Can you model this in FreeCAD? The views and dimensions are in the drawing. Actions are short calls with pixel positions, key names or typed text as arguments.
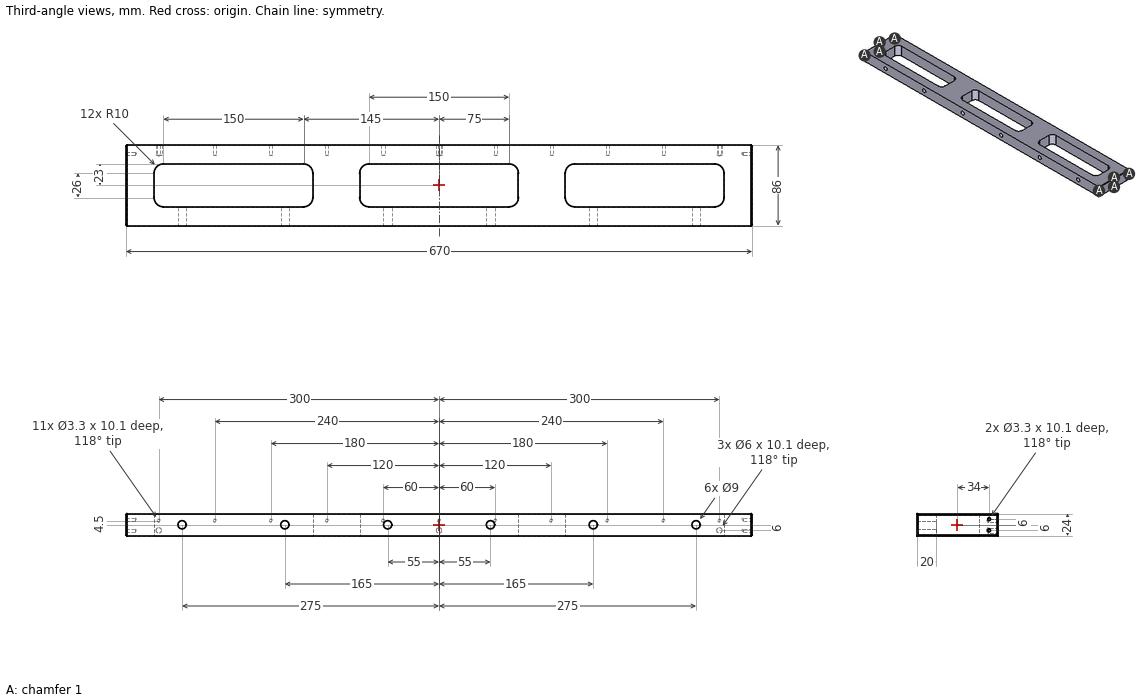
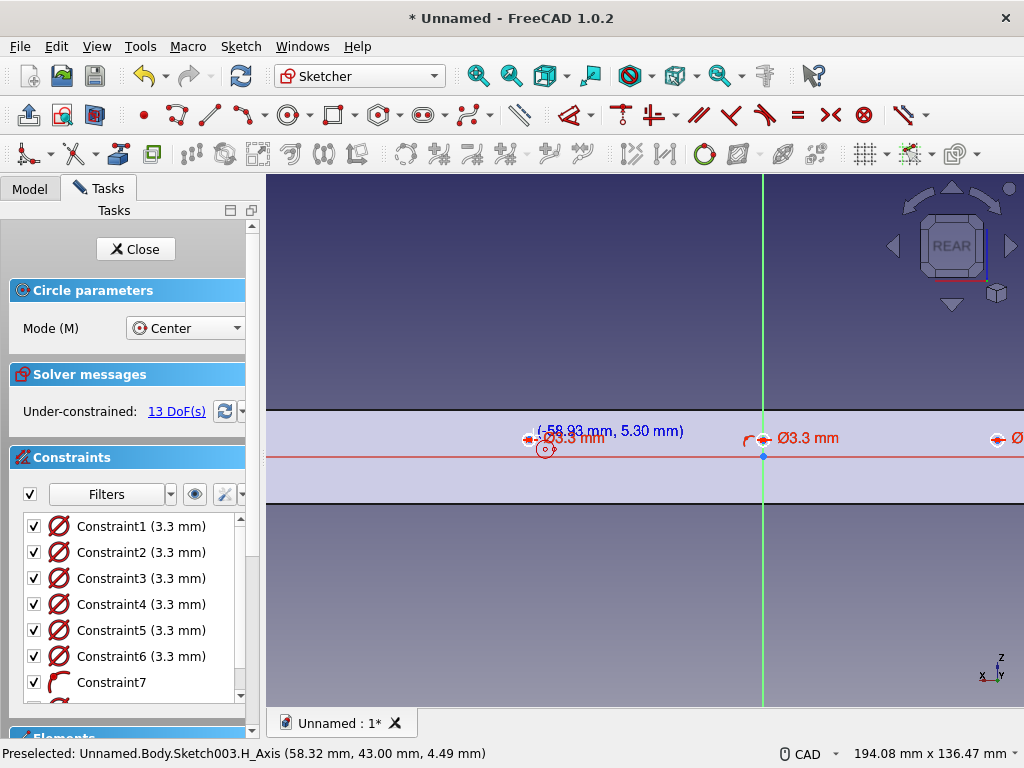
scroll(294, 439, up, 7)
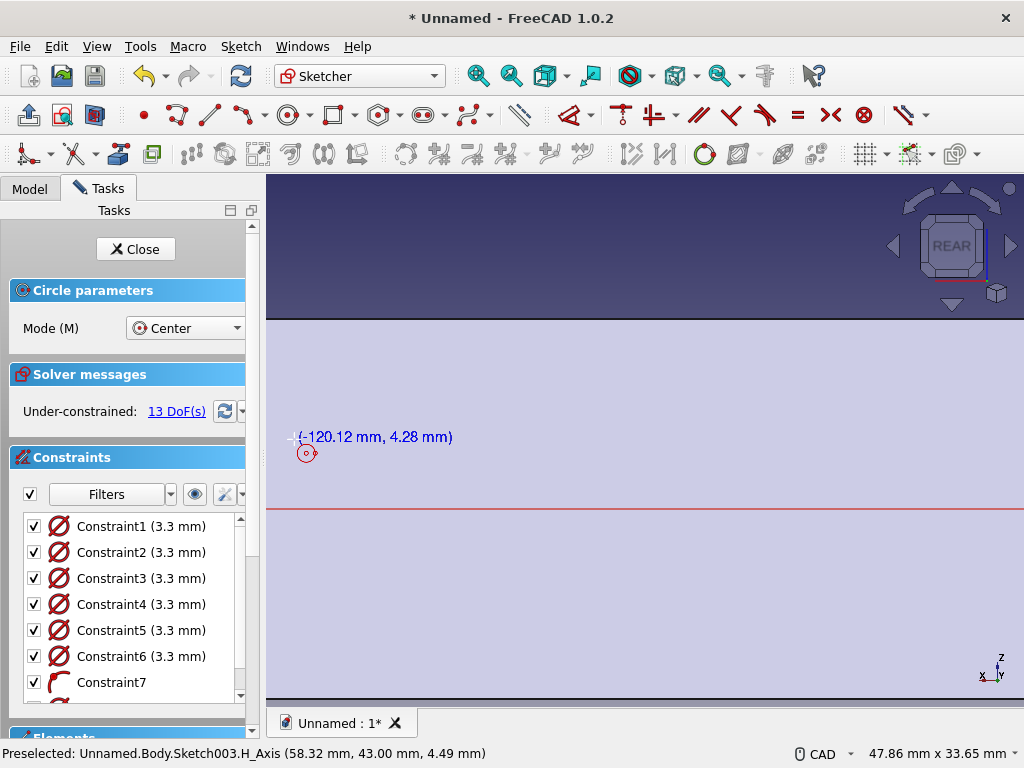
scroll(492, 439, down, 15)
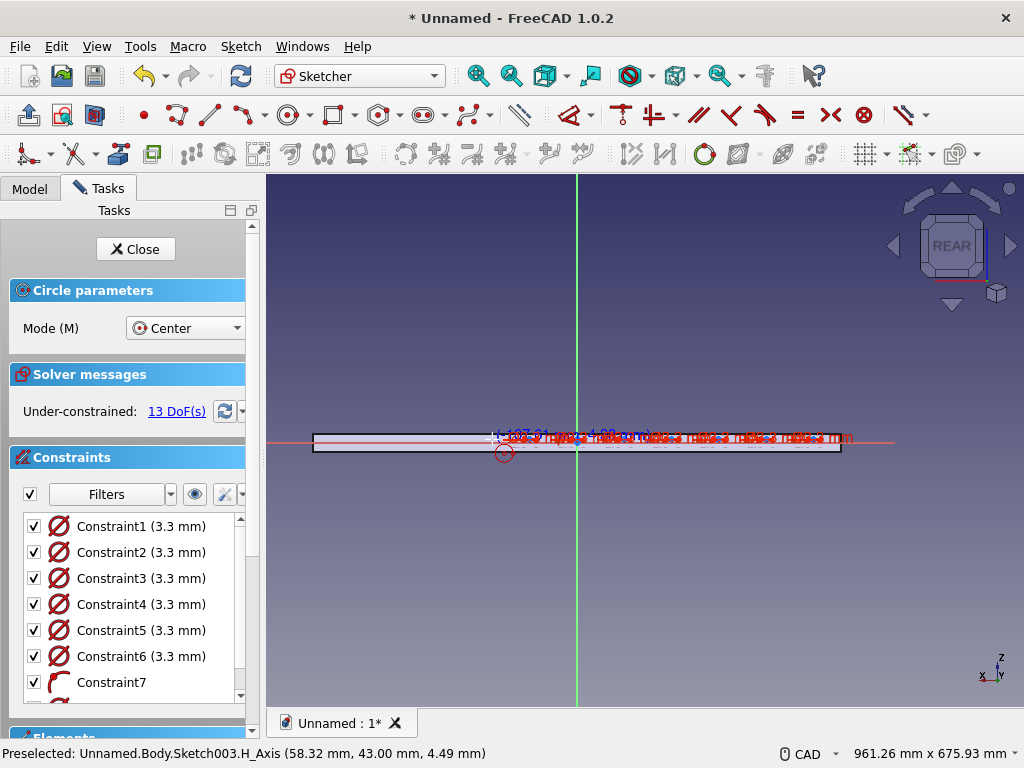
scroll(483, 439, up, 8)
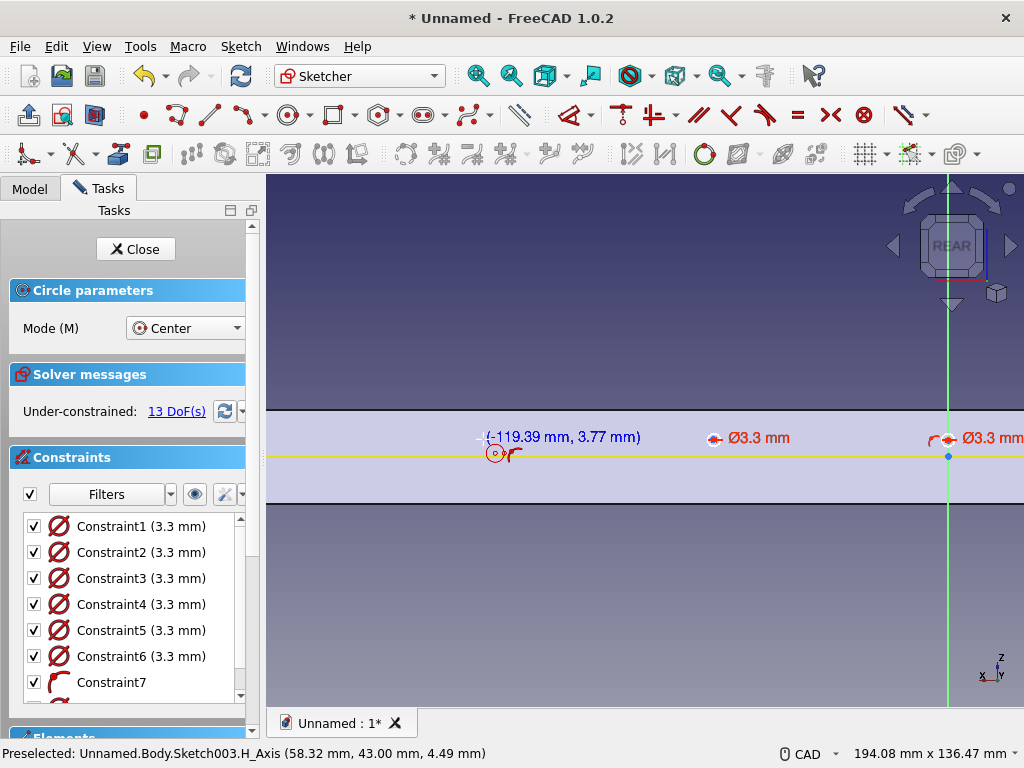
click(479, 439)
move(484, 435)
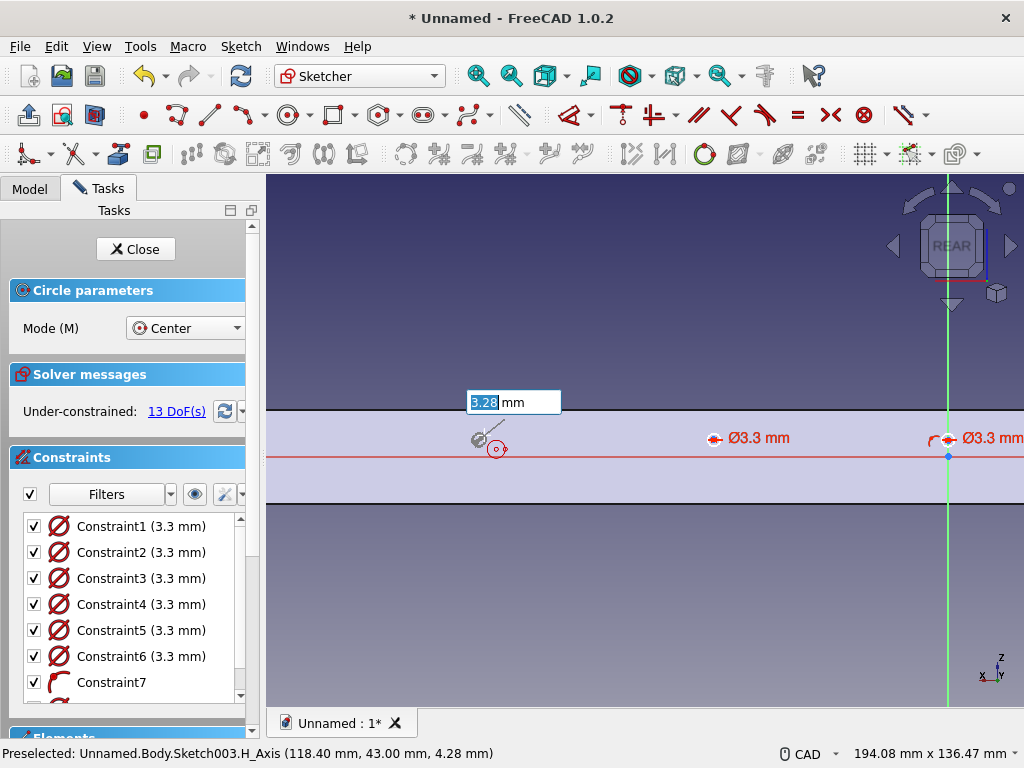
text(3.3)
key(Return)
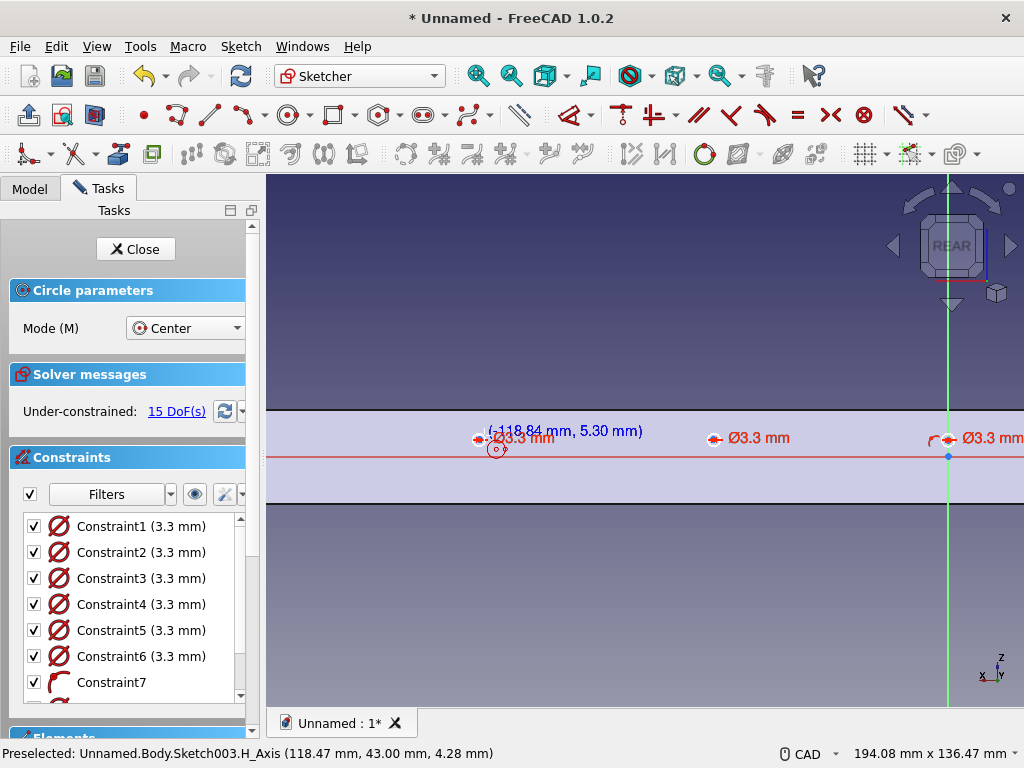
scroll(503, 440, down, 9)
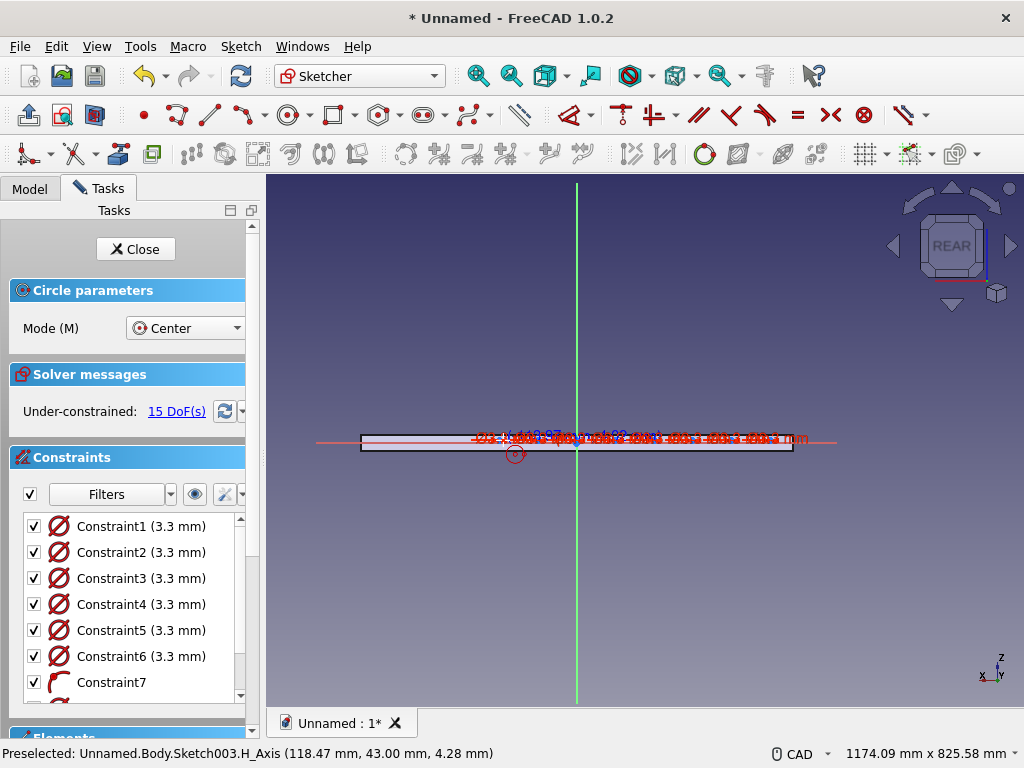
scroll(461, 440, up, 16)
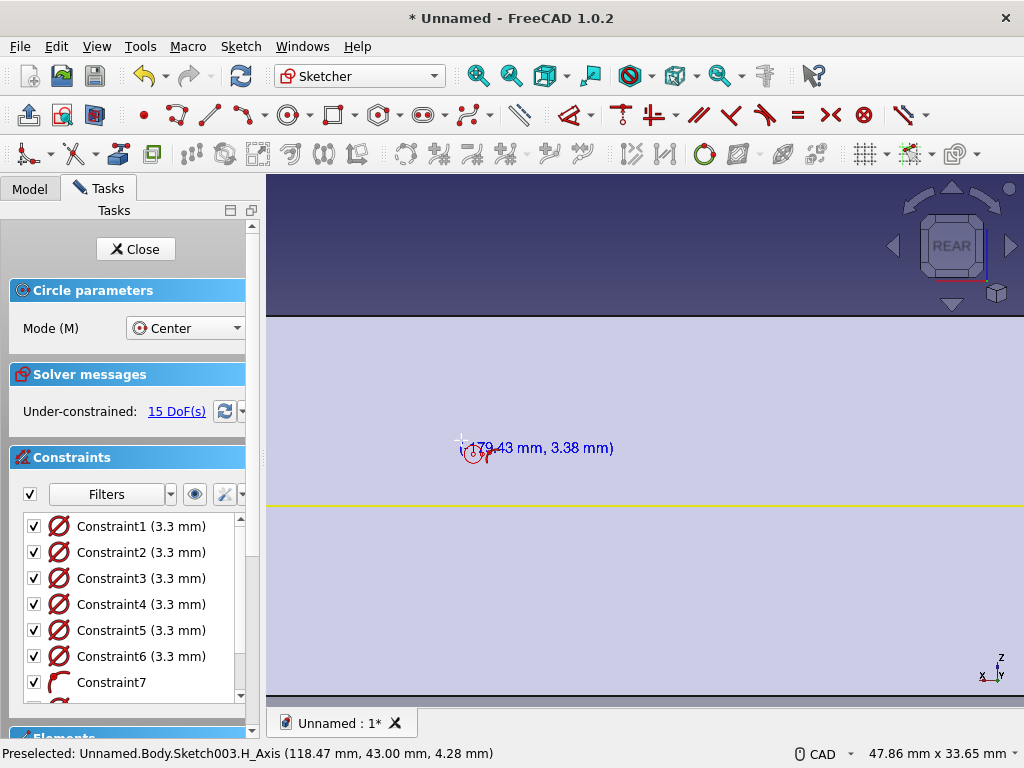
scroll(434, 440, down, 15)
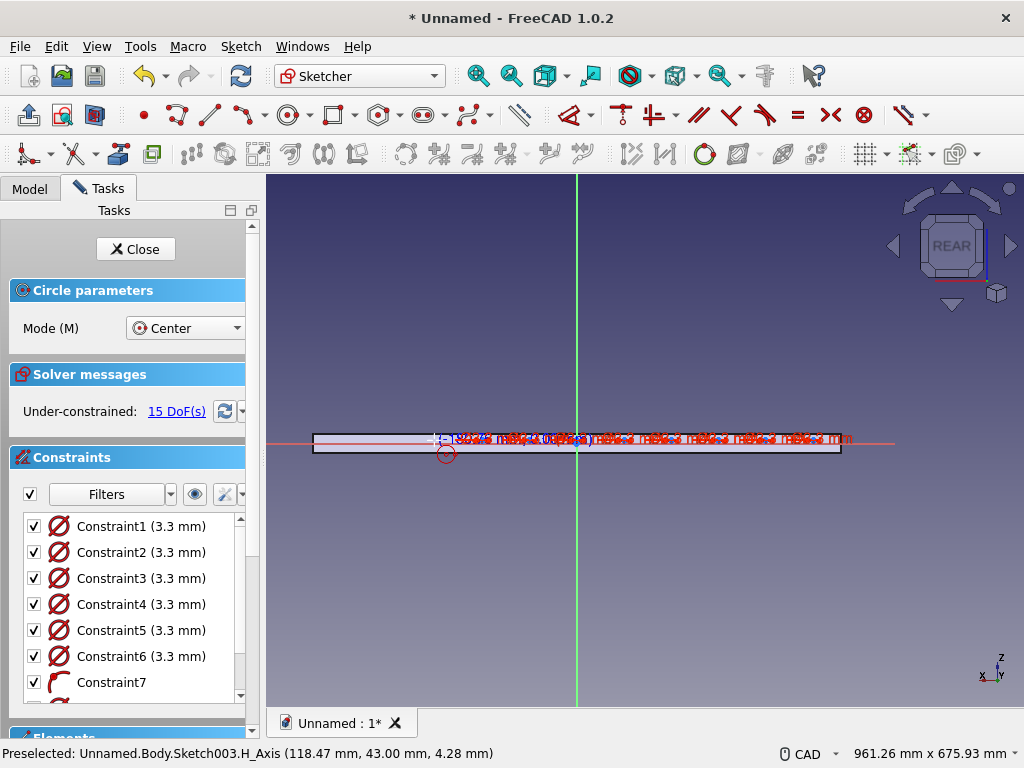
scroll(435, 440, up, 8)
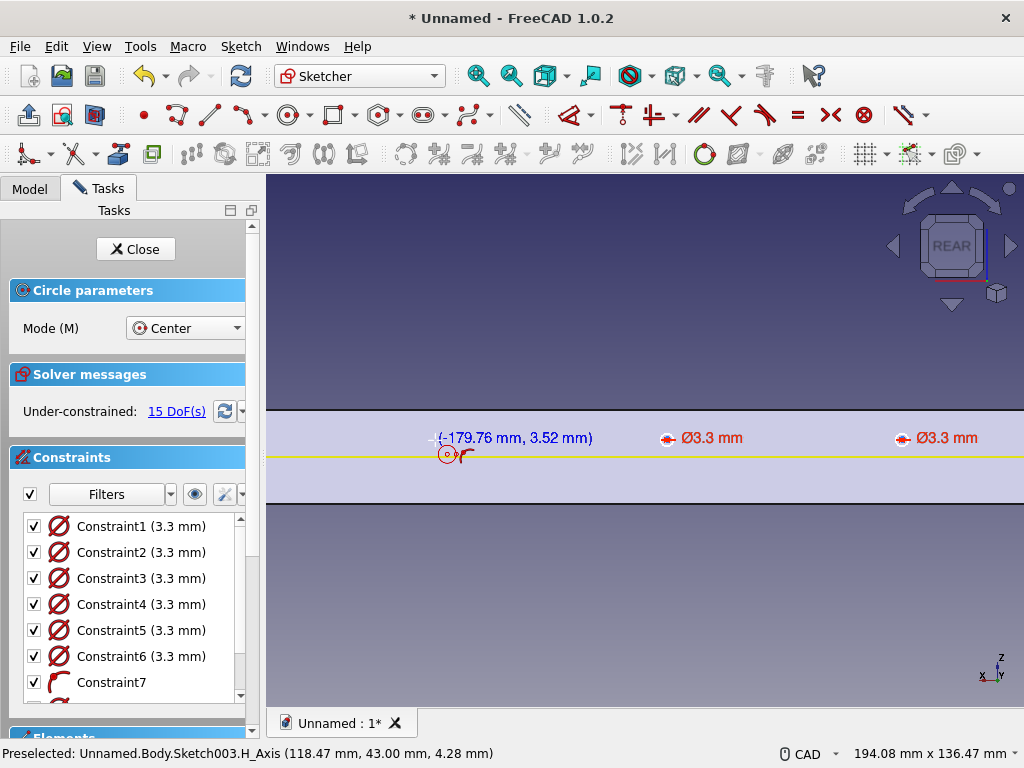
click(433, 439)
move(438, 435)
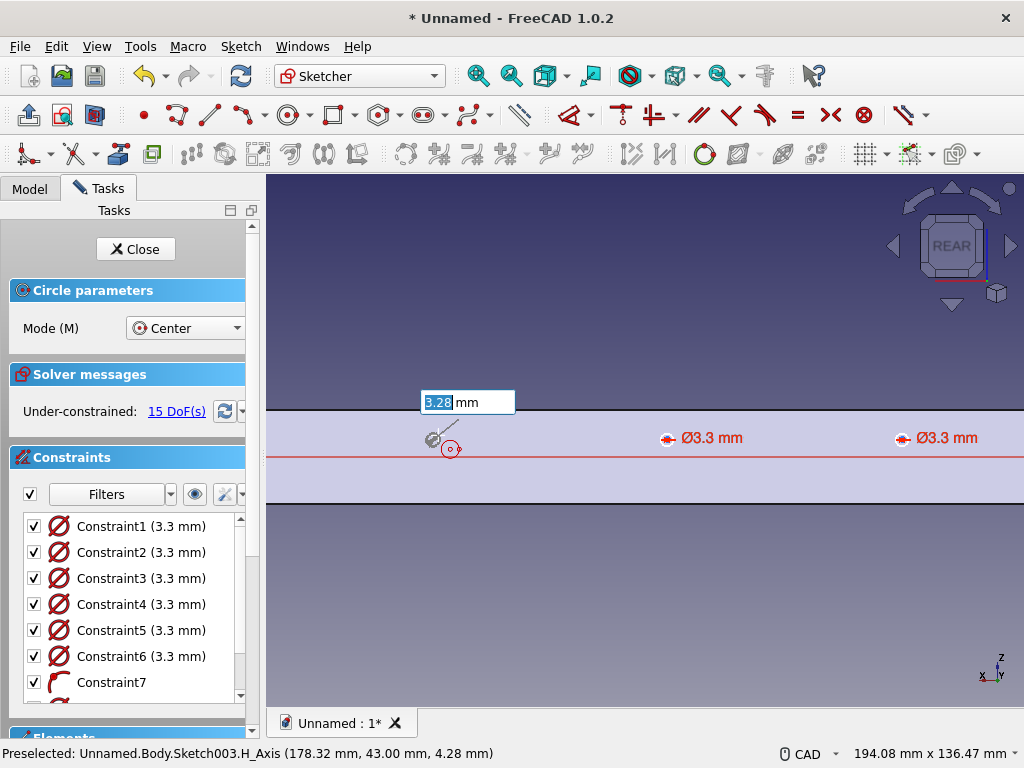
text(3.3)
key(Return)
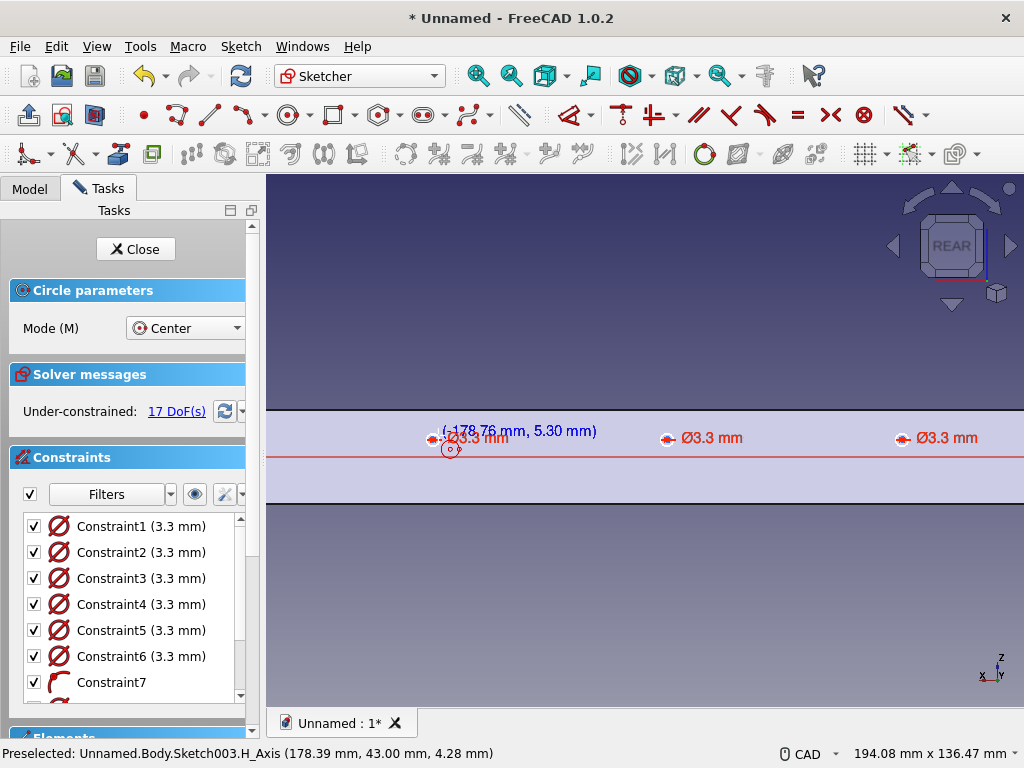
scroll(466, 440, down, 9)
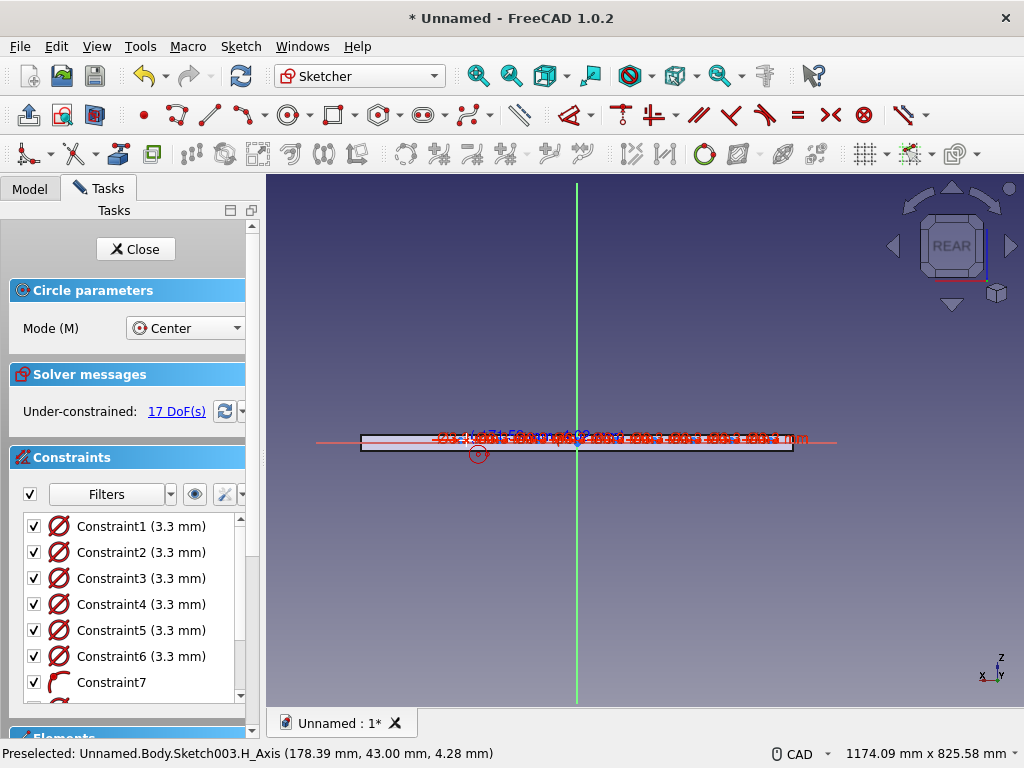
scroll(422, 440, up, 16)